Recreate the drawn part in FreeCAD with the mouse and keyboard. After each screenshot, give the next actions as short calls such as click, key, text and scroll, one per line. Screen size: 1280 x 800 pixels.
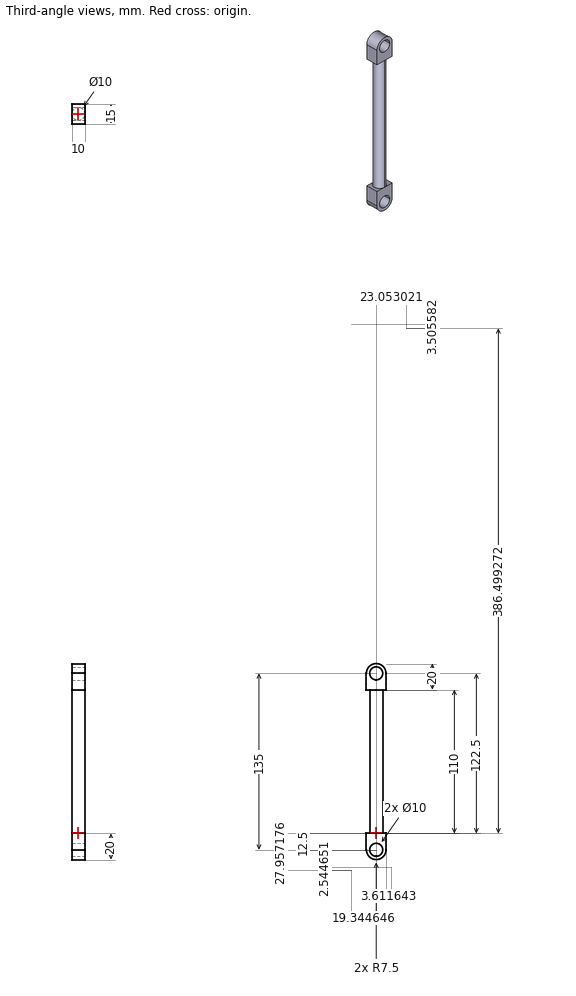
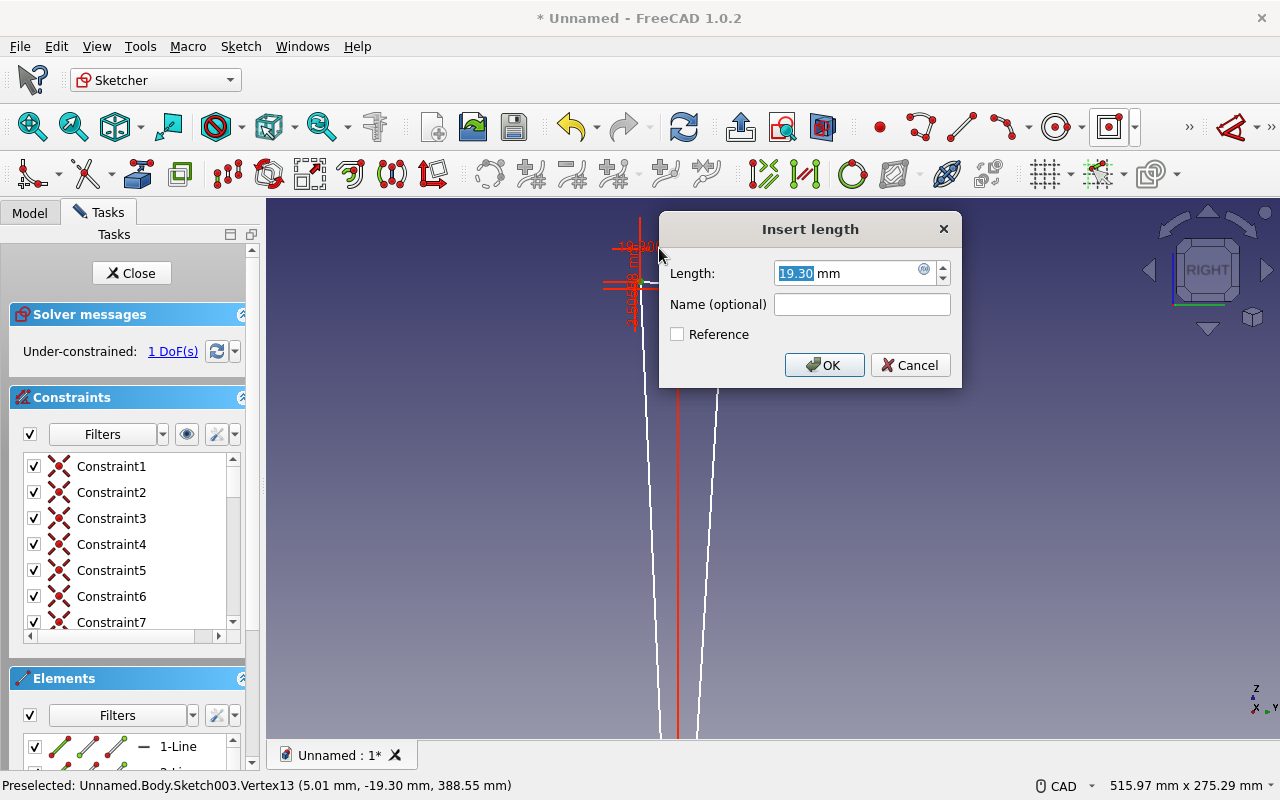
text(19.344646)
key(Return)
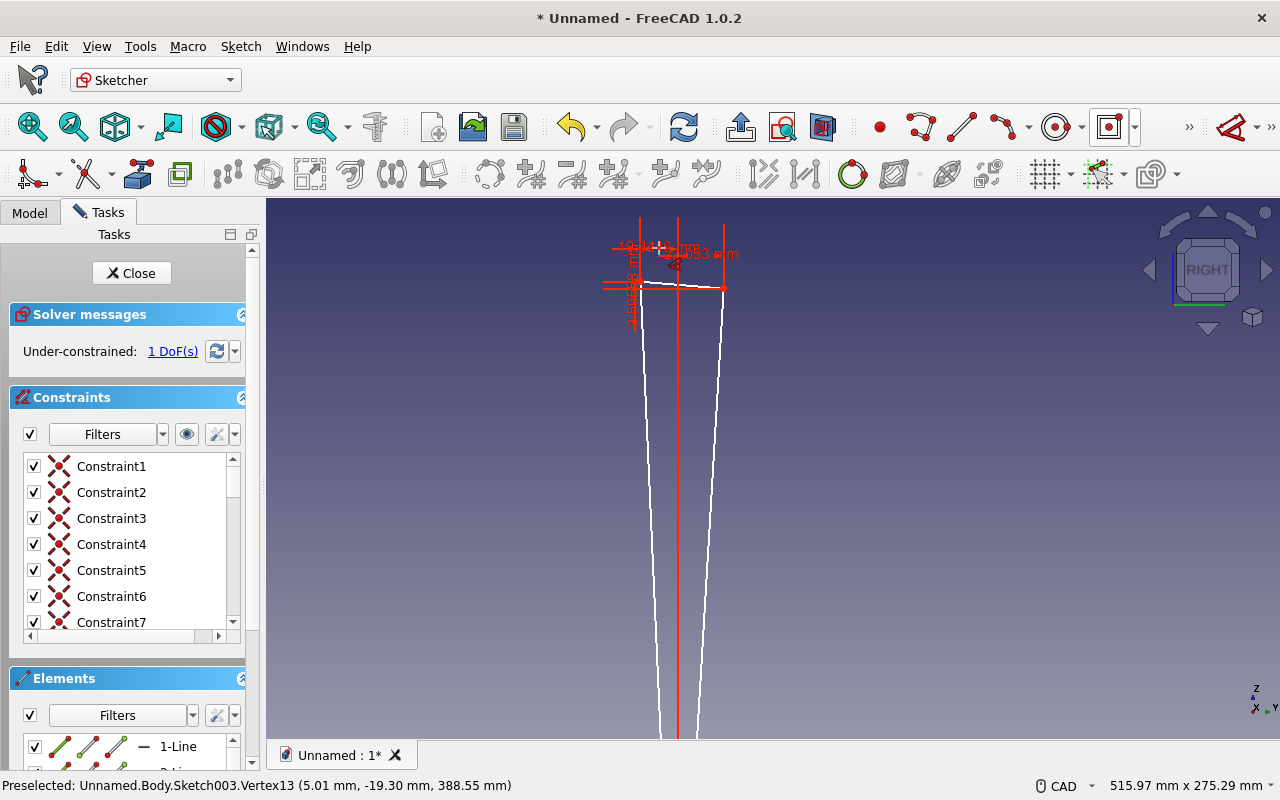
click(724, 289)
click(758, 500)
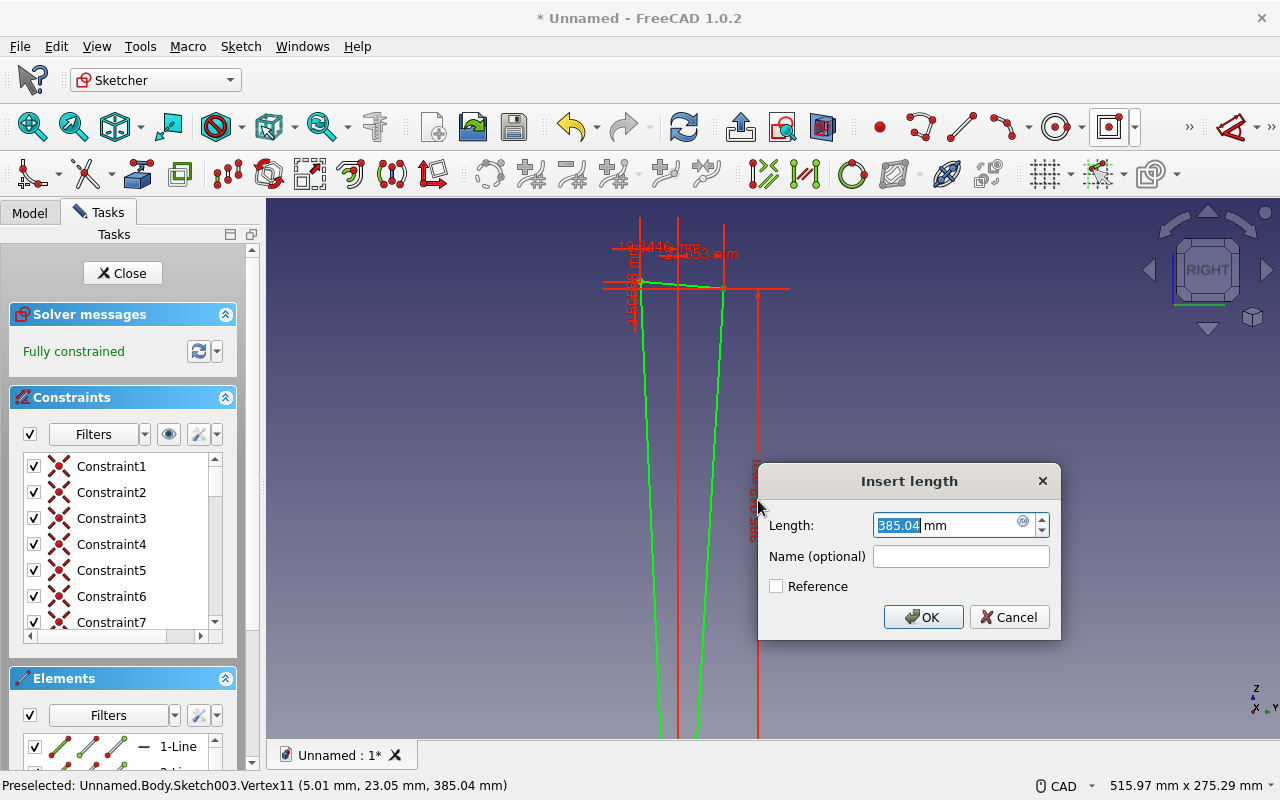
text(386.499272)
key(Return)
key(Escape)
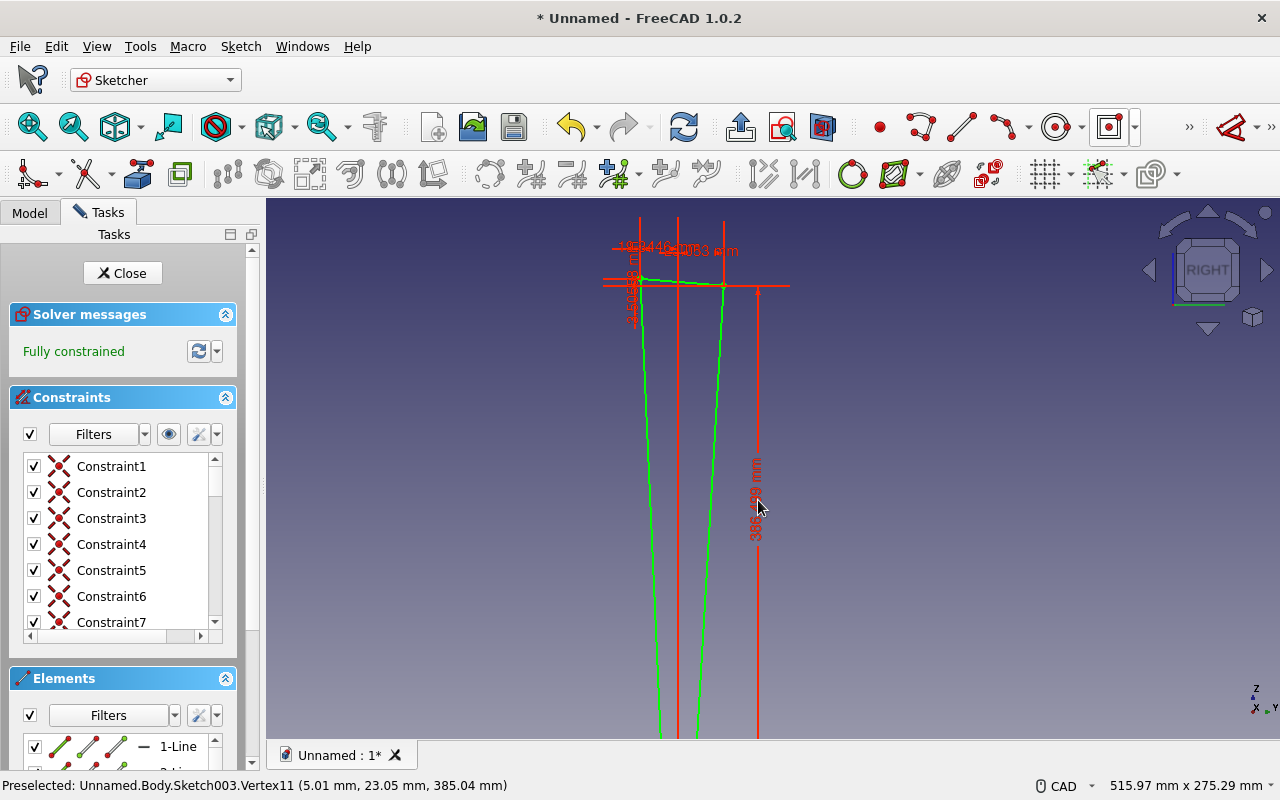
click(123, 273)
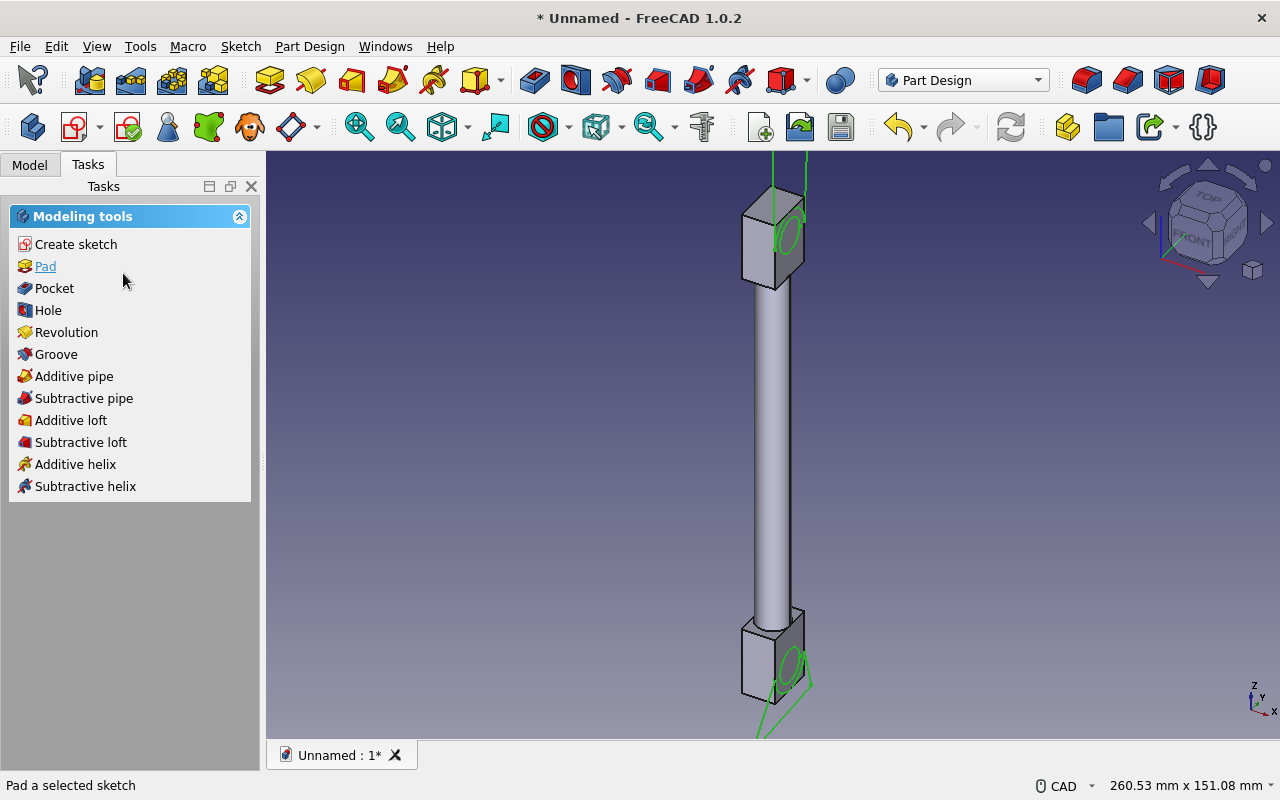
click(535, 80)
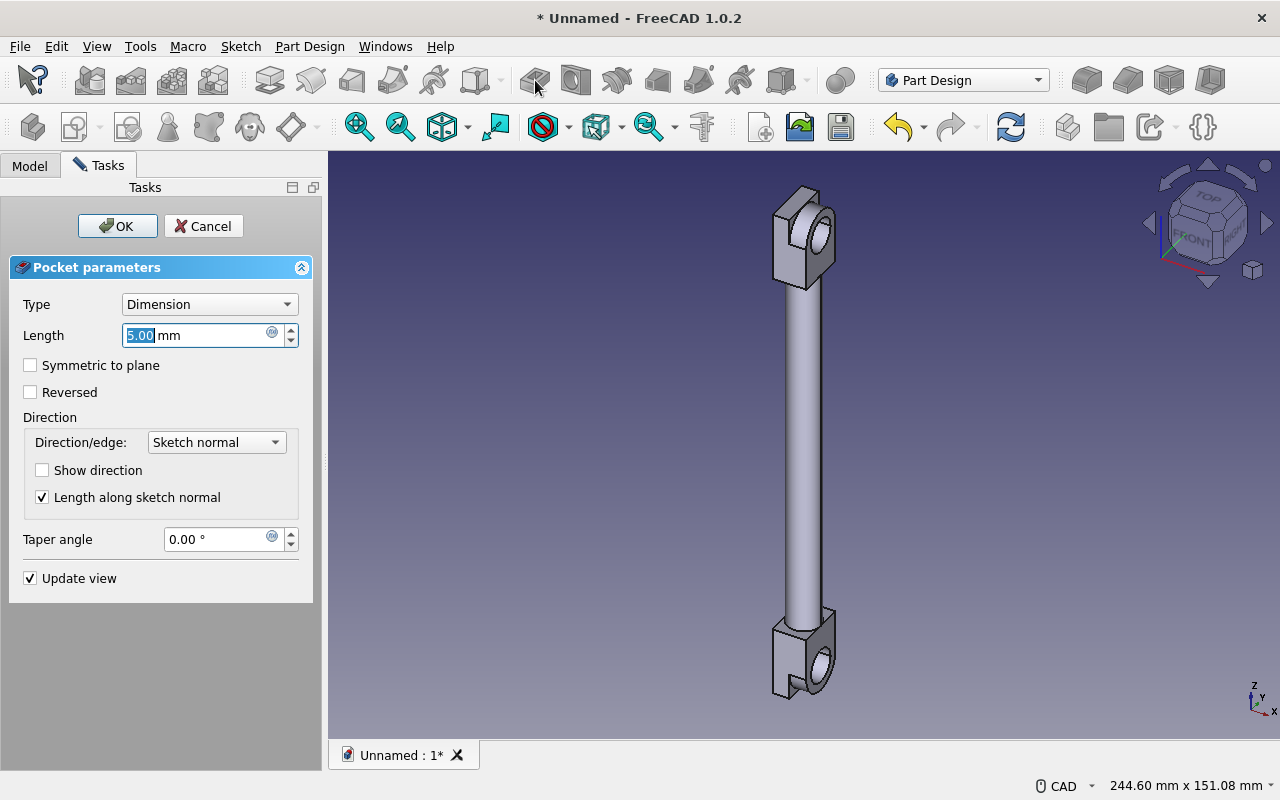
click(210, 304)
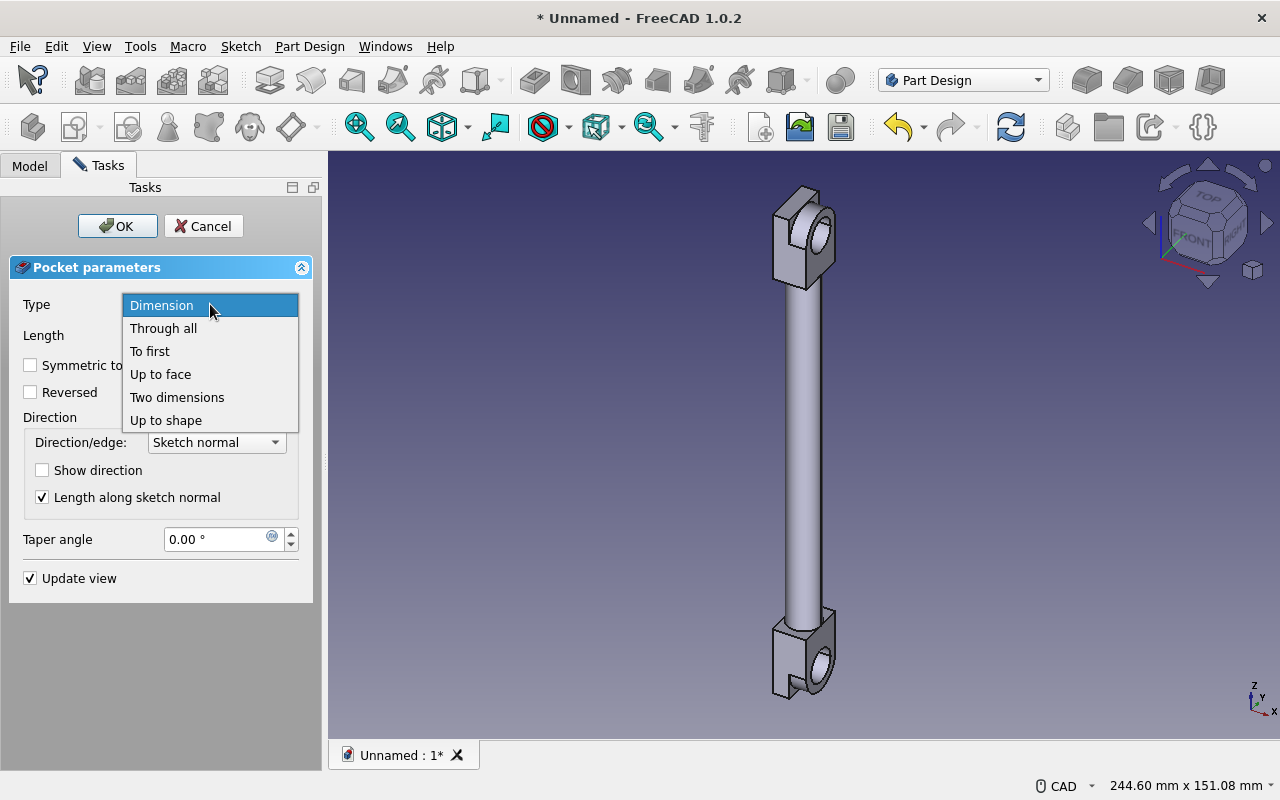
click(208, 328)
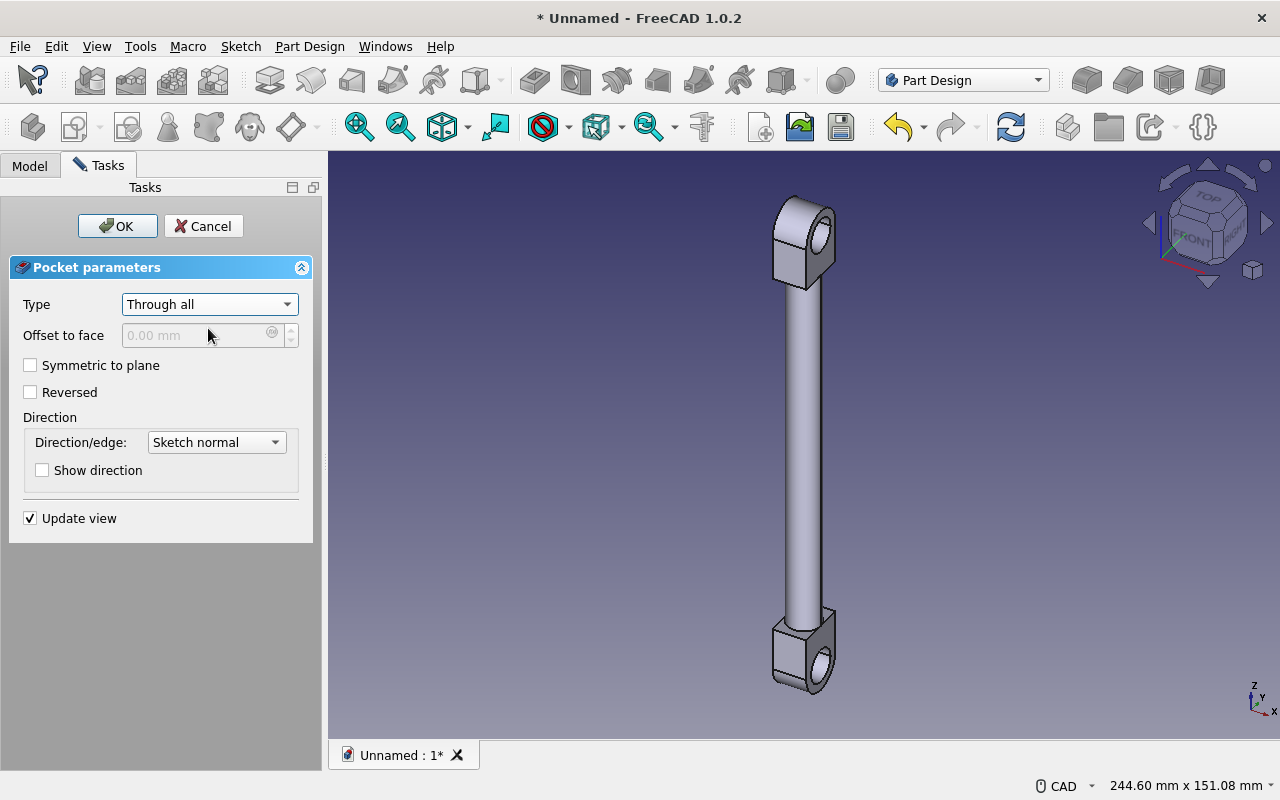
click(118, 226)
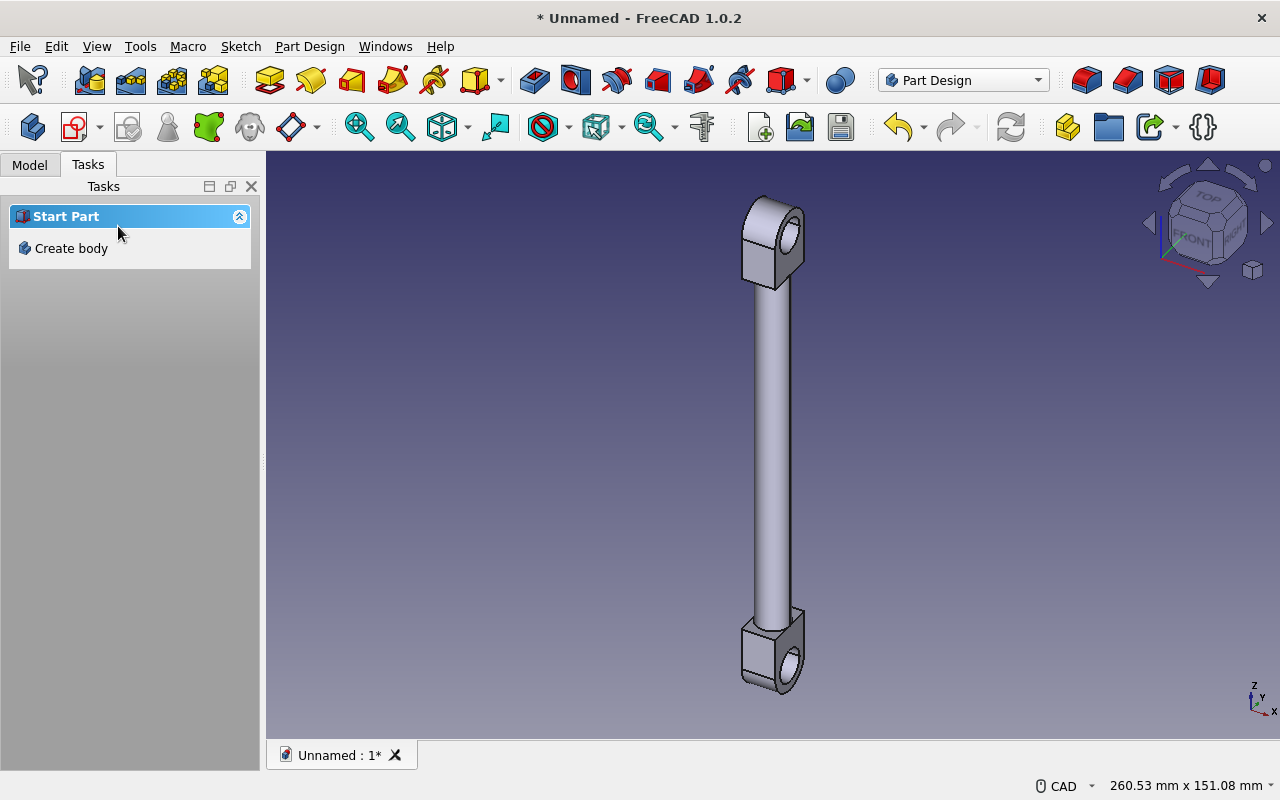
key(0)